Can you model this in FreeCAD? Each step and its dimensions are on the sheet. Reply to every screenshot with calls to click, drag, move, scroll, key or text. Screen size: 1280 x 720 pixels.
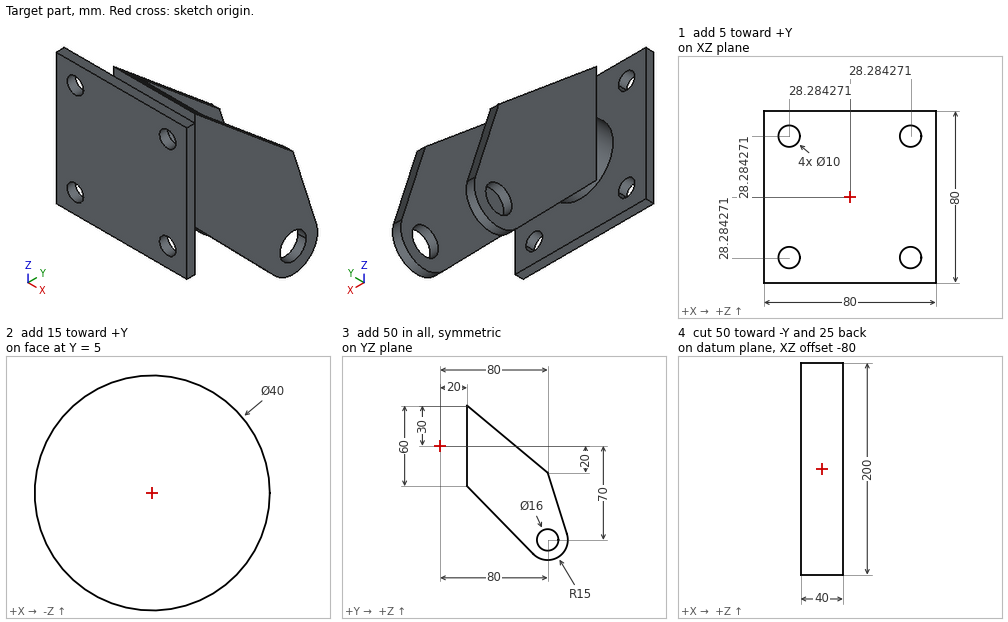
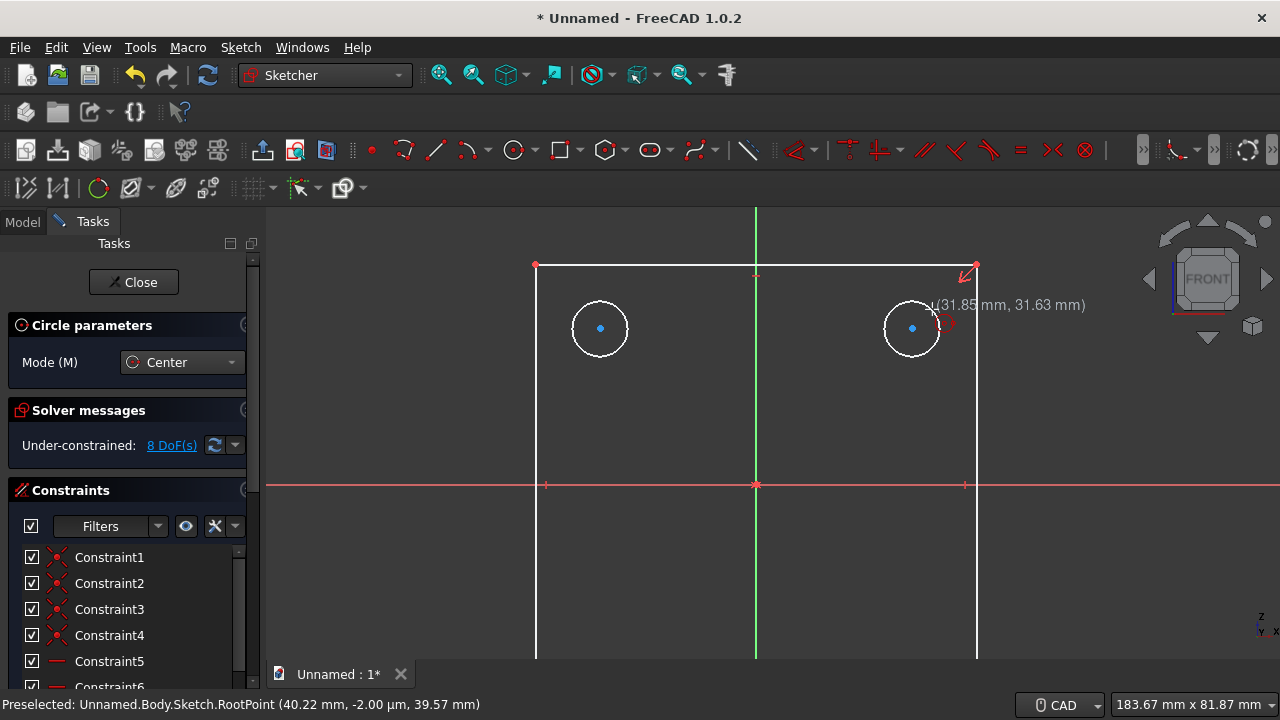
scroll(599, 328, down, 2)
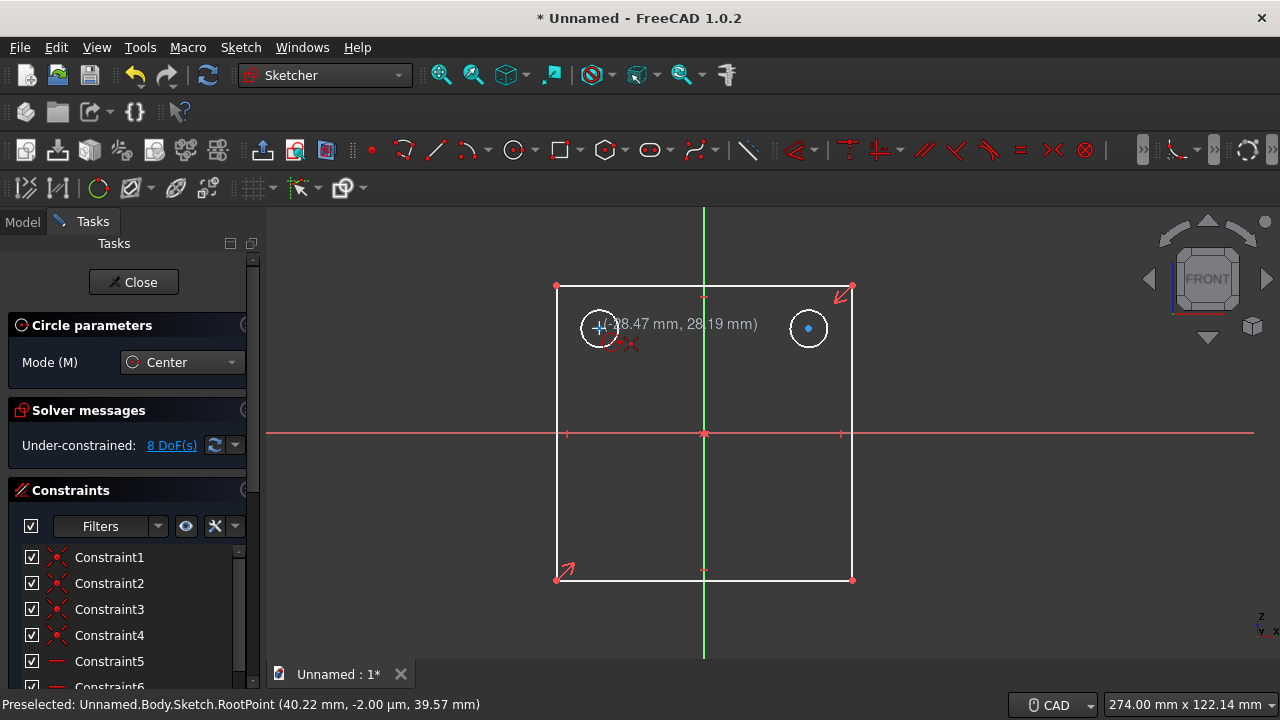
scroll(600, 538, up, 2)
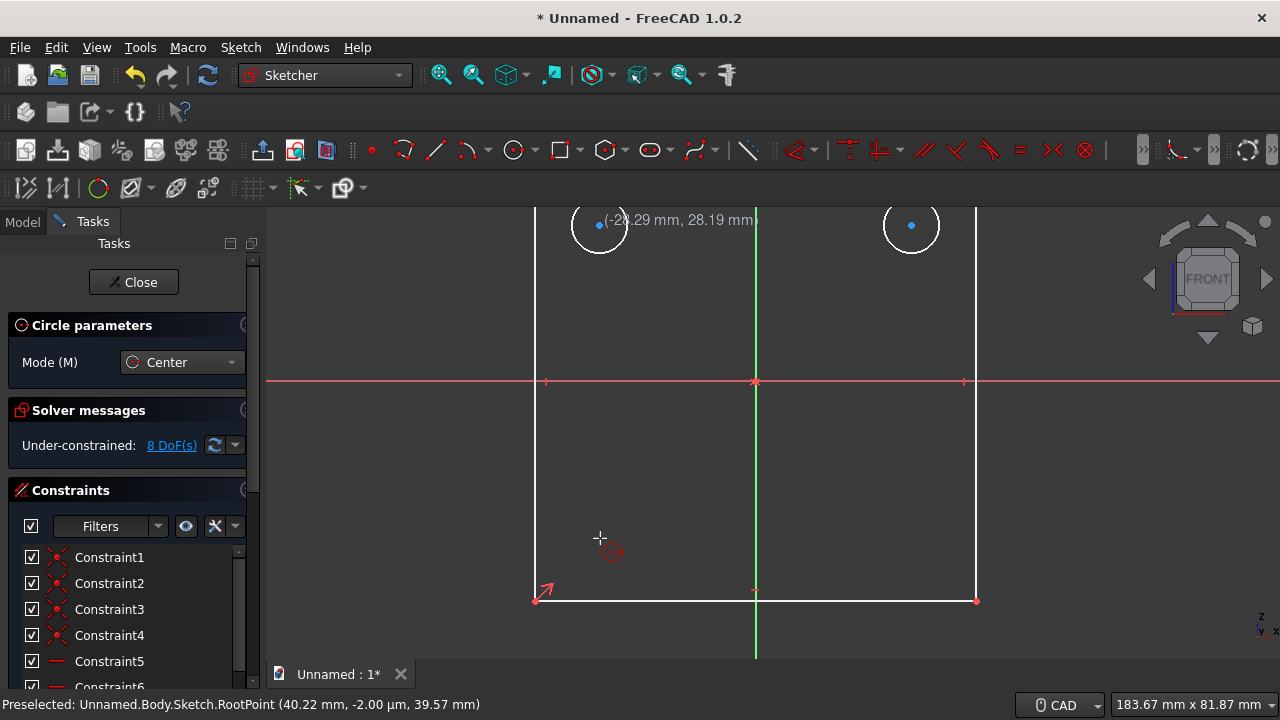
click(600, 537)
click(619, 518)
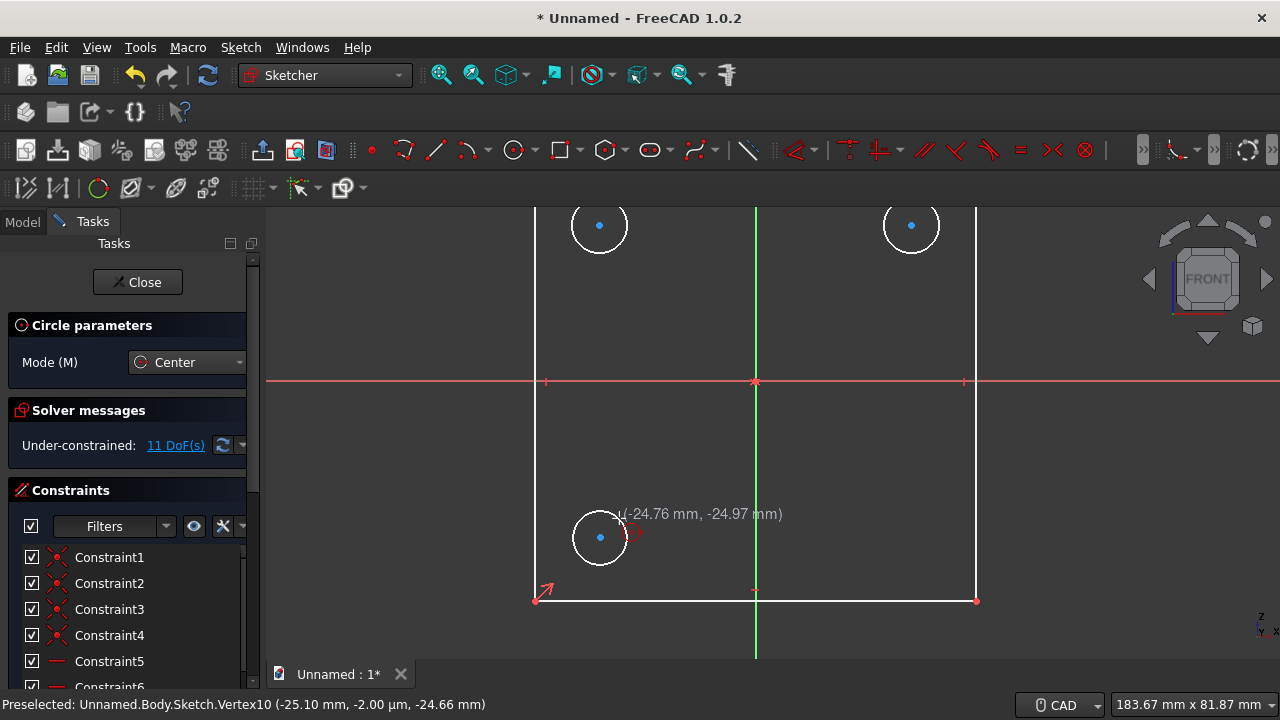
click(912, 537)
click(931, 518)
key(Escape)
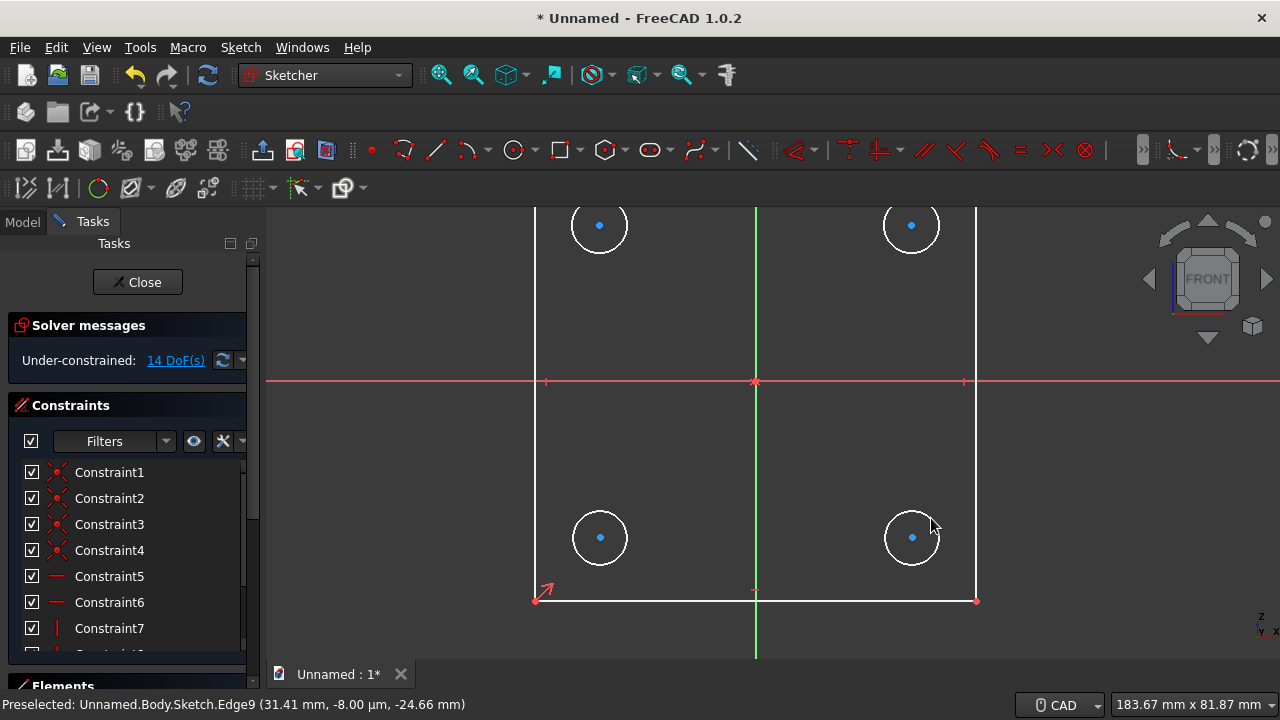
click(580, 245)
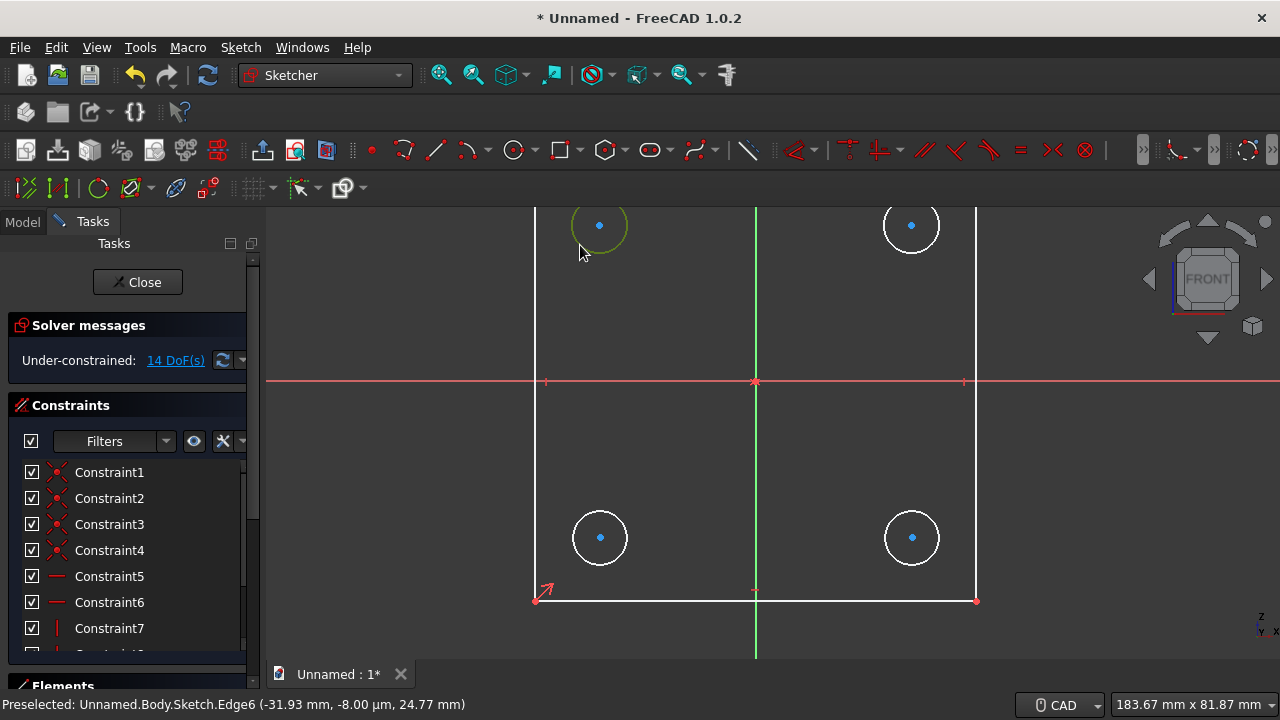
click(892, 245)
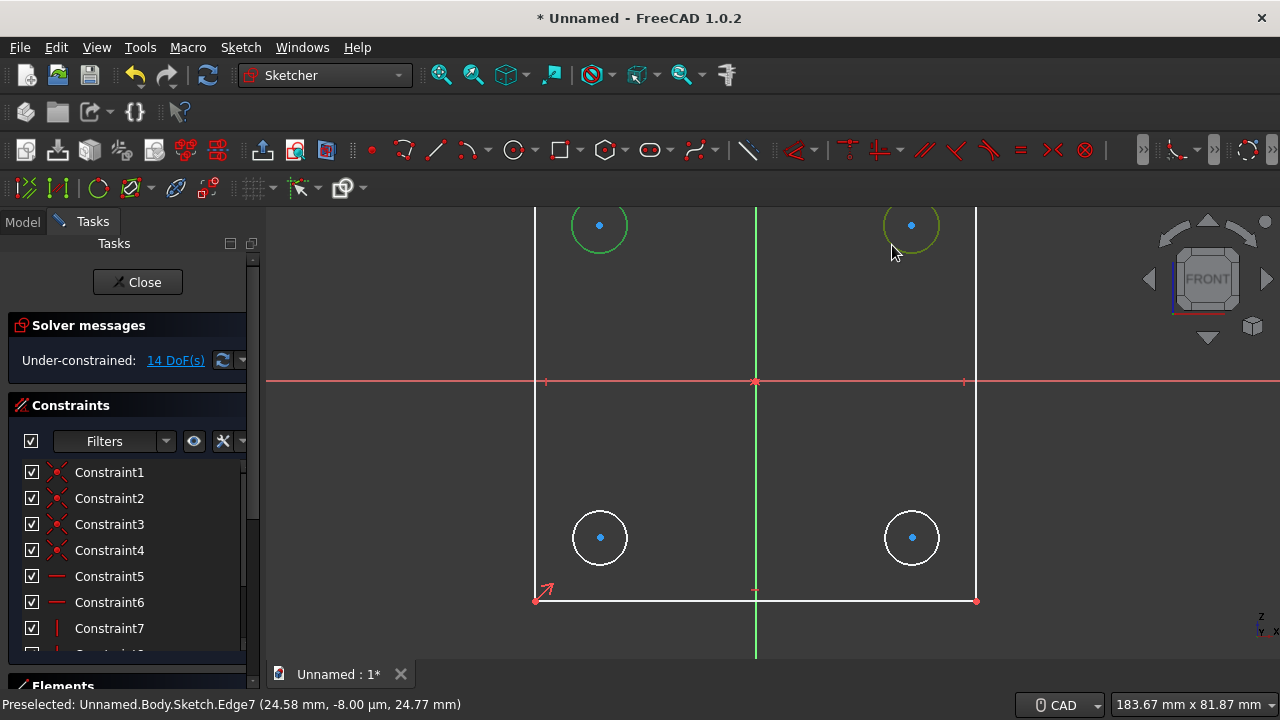
click(619, 519)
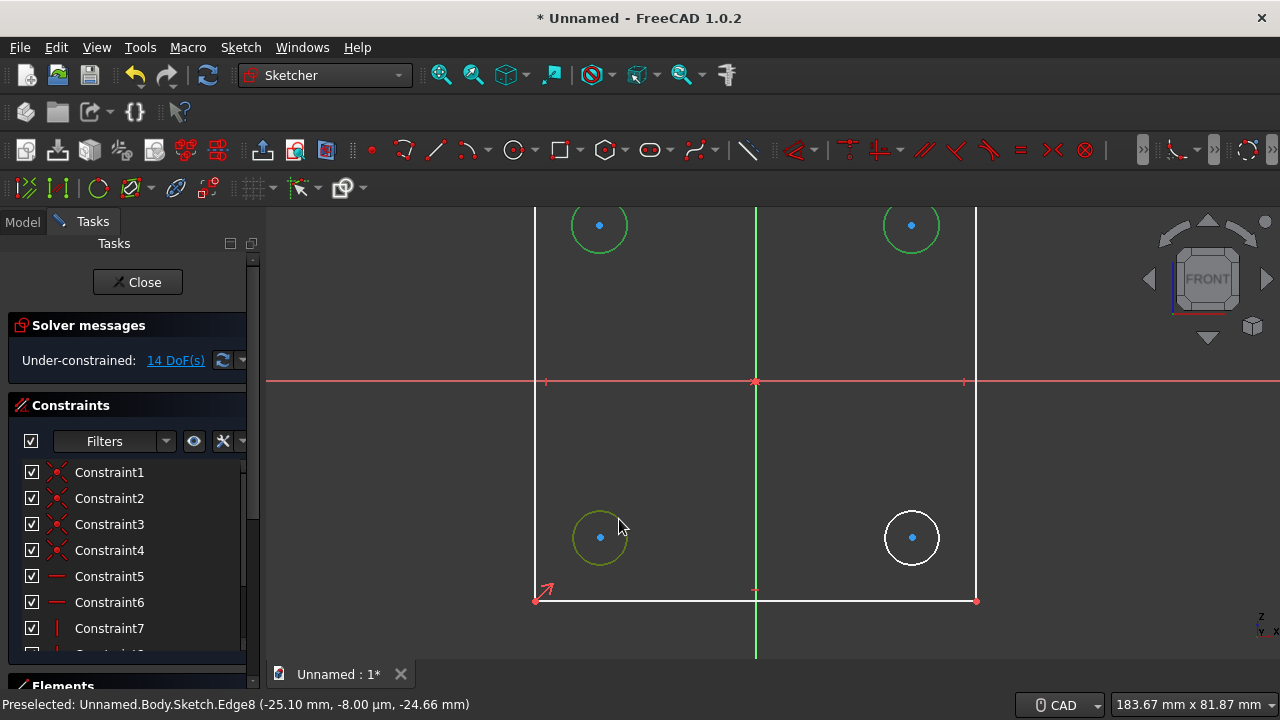
click(931, 519)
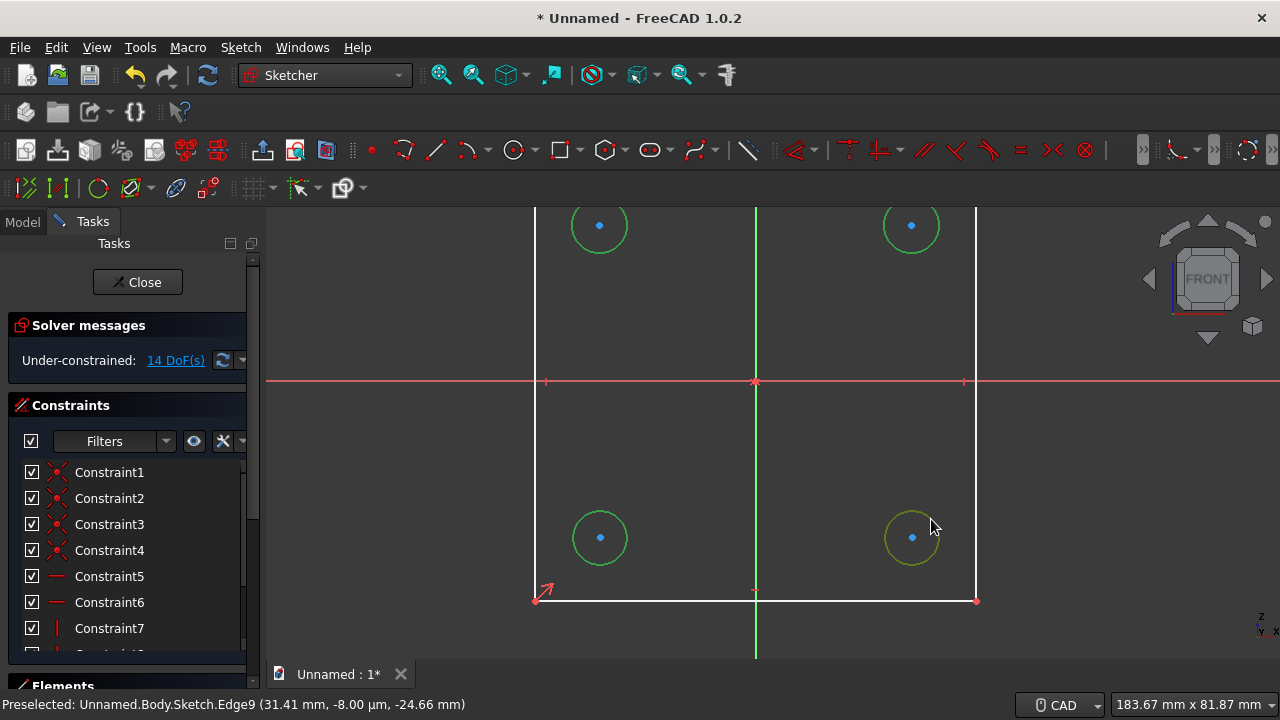
click(1022, 150)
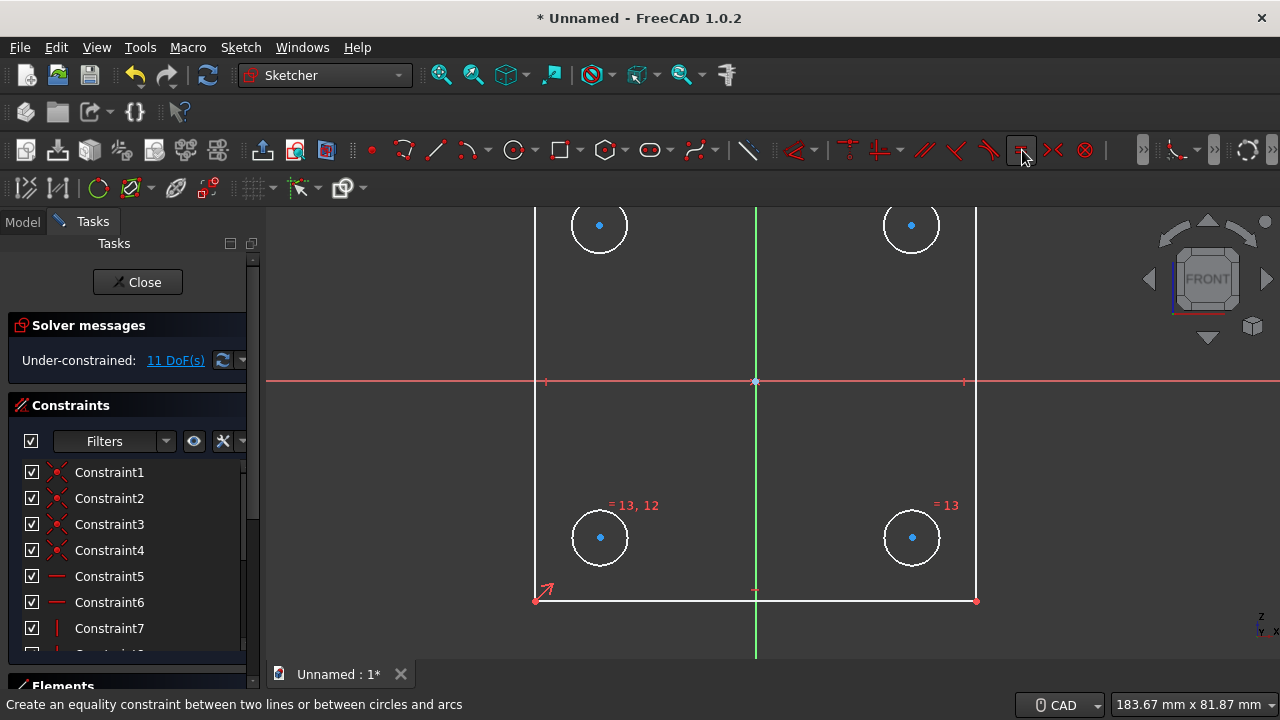
scroll(600, 538, down, 2)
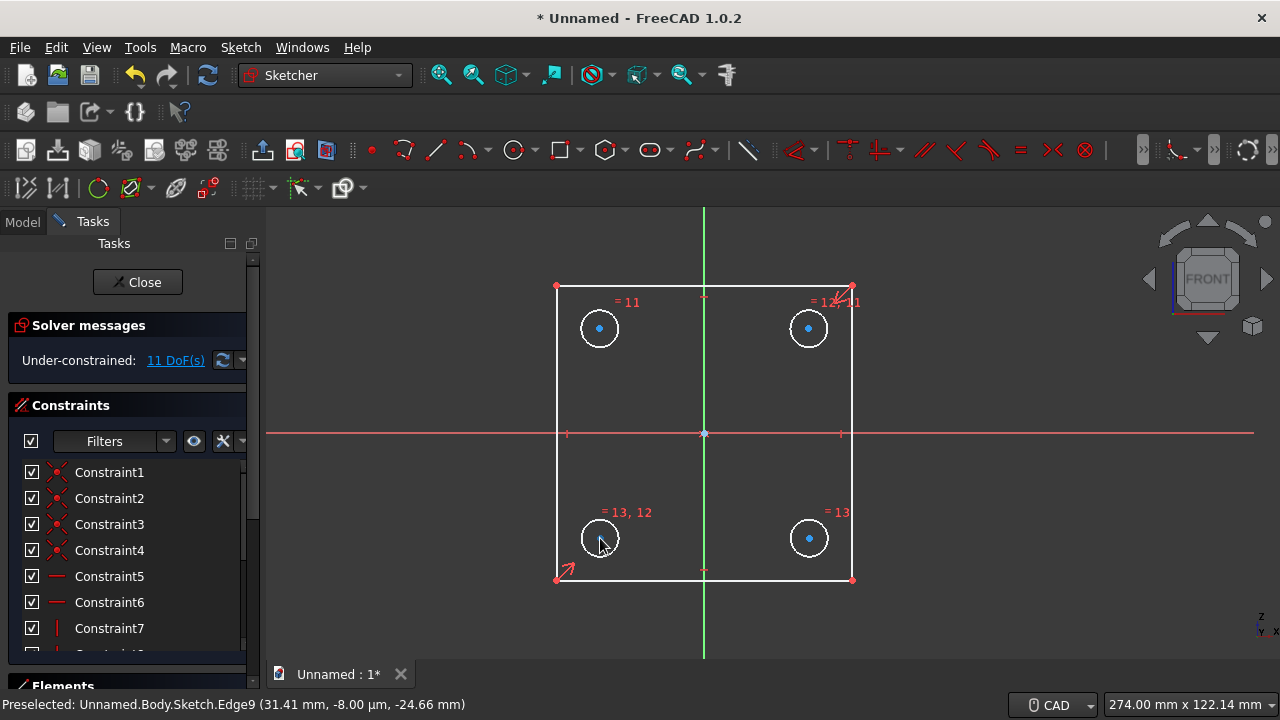
click(600, 329)